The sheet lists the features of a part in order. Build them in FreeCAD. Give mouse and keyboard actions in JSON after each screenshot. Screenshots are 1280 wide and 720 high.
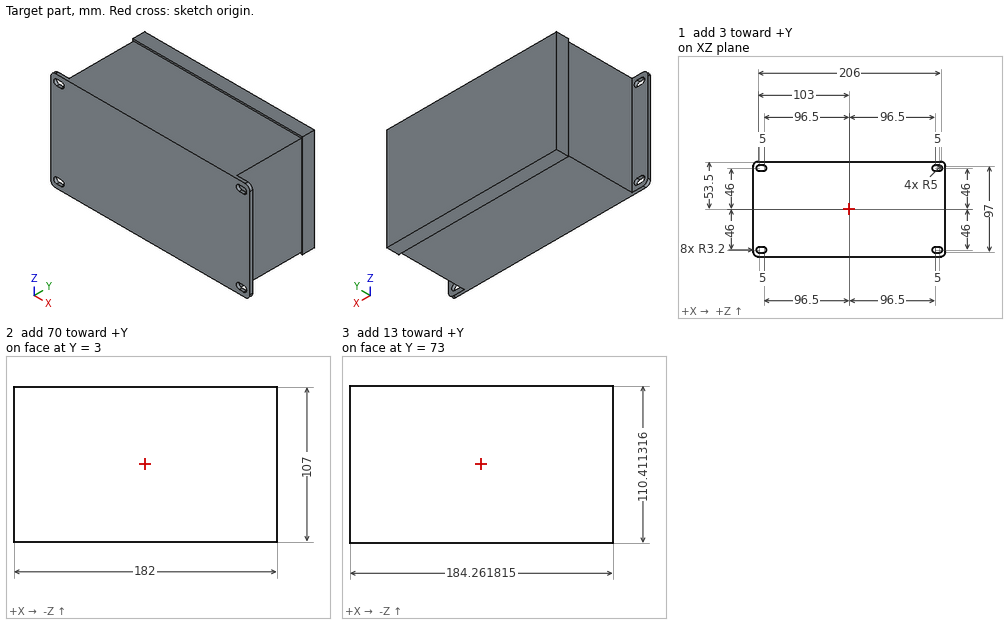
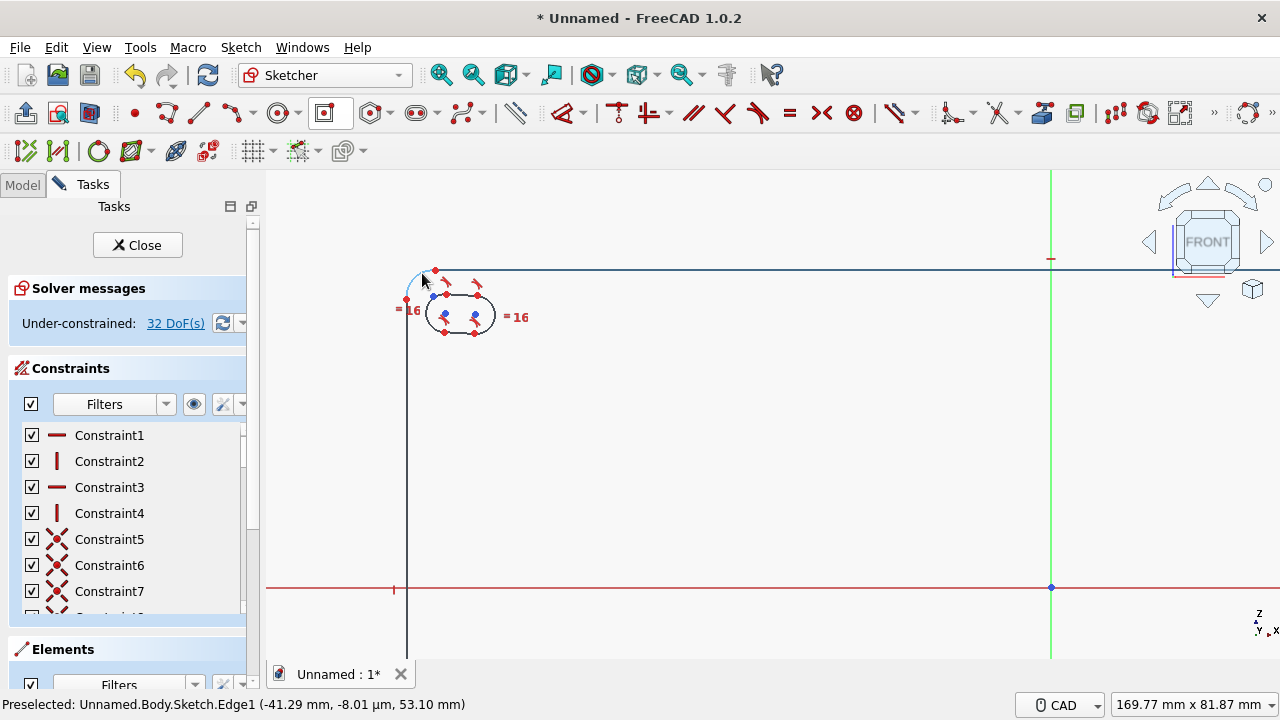
{"action": "left_click", "coordinate": [422, 273]}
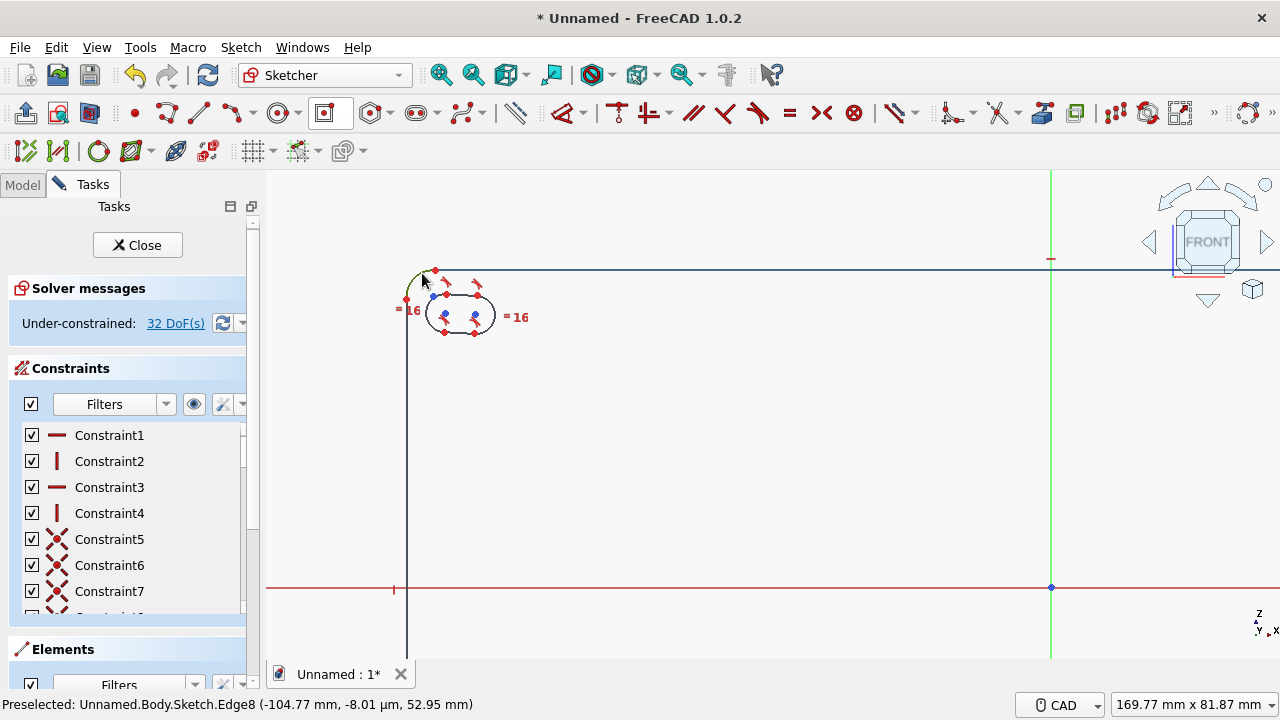
{"action": "left_click", "coordinate": [758, 114]}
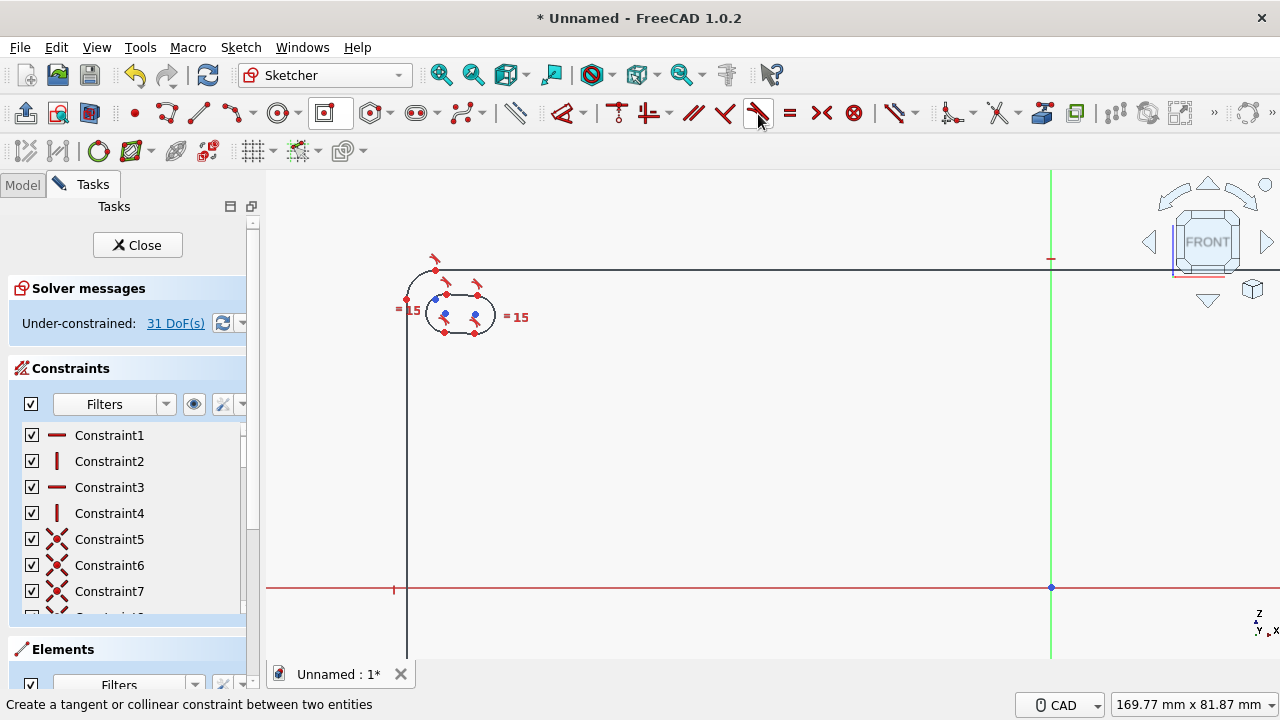
{"action": "scroll", "coordinate": [421, 273], "scroll_direction": "down", "scroll_amount": 4}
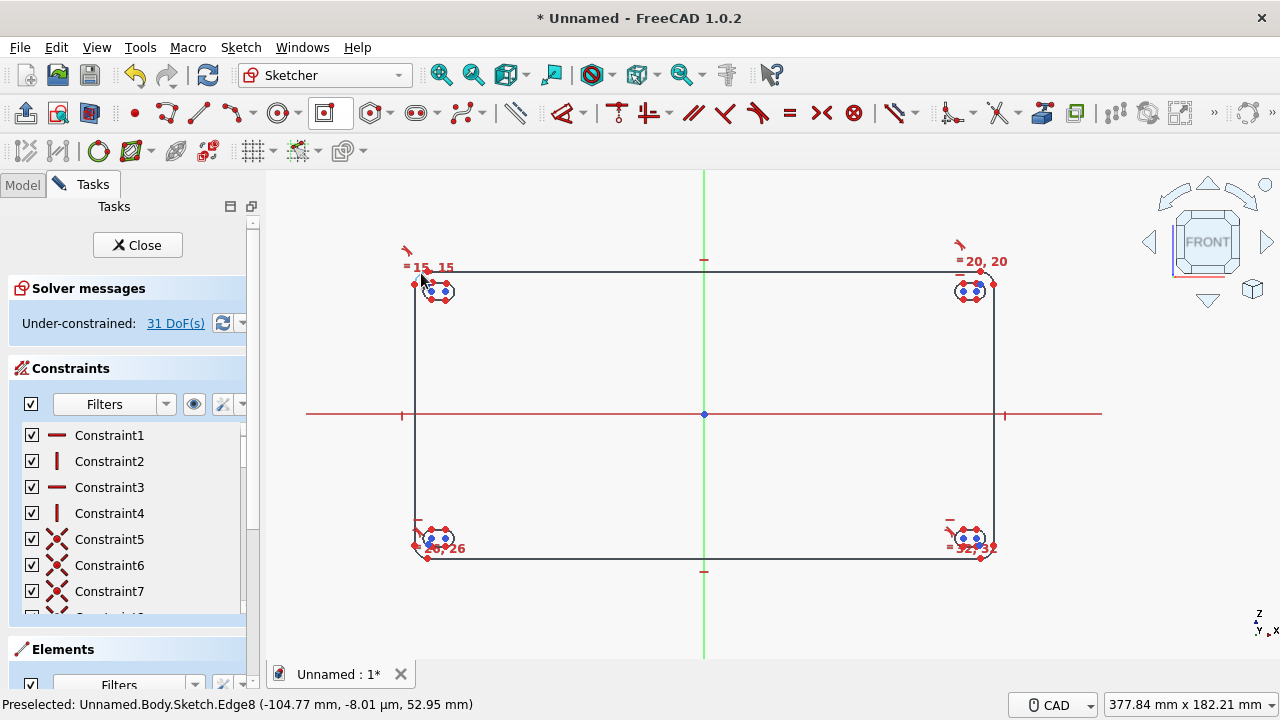
{"action": "left_click", "coordinate": [994, 363]}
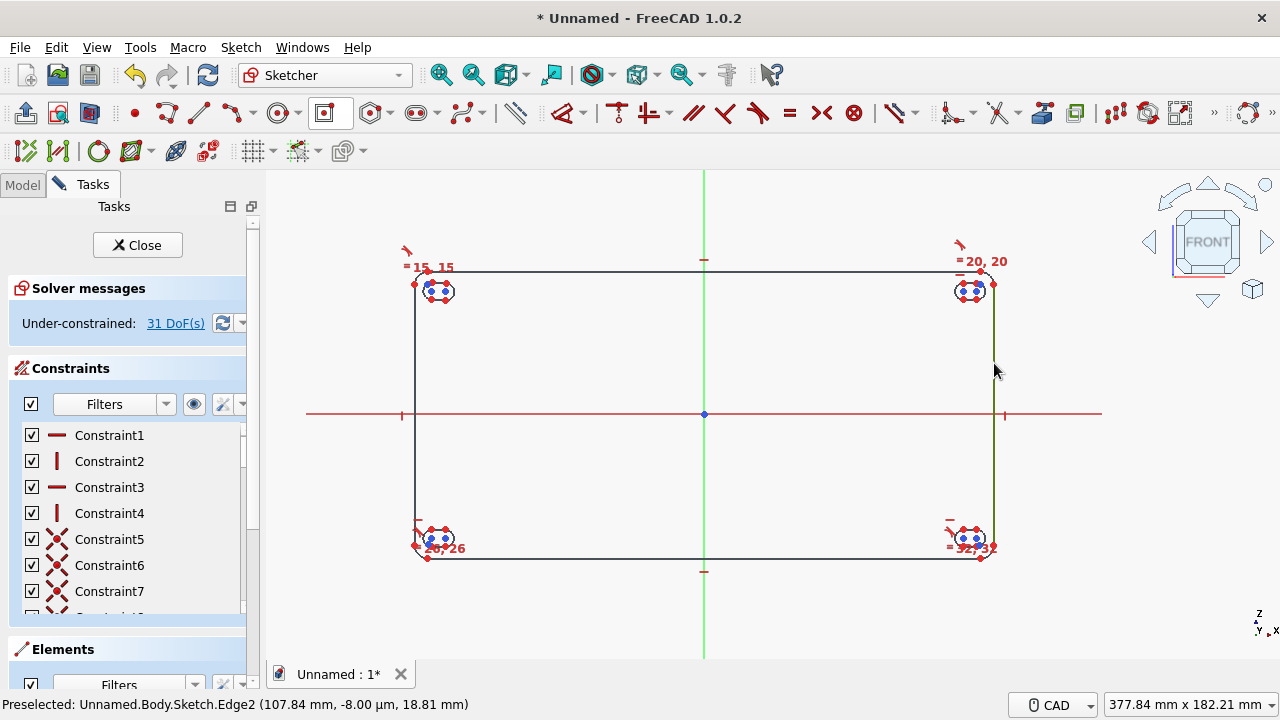
{"action": "scroll", "coordinate": [990, 276], "scroll_direction": "up", "scroll_amount": 2}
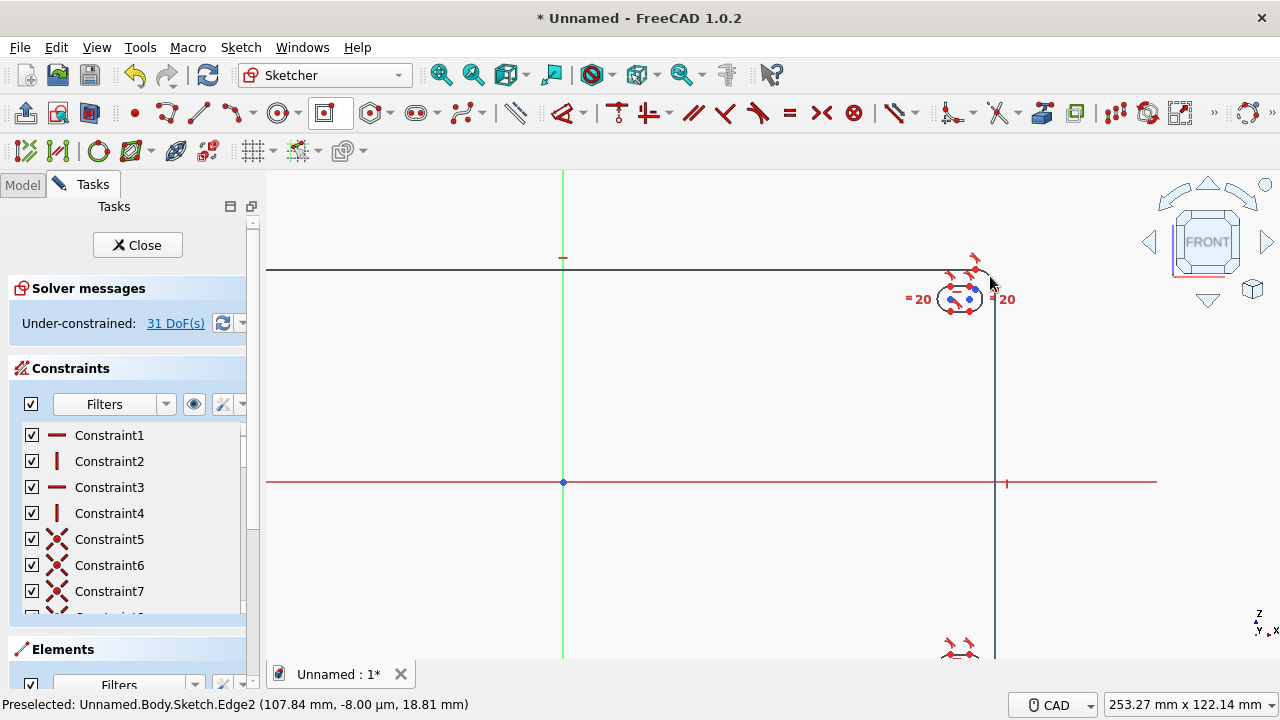
{"action": "left_click", "coordinate": [990, 276]}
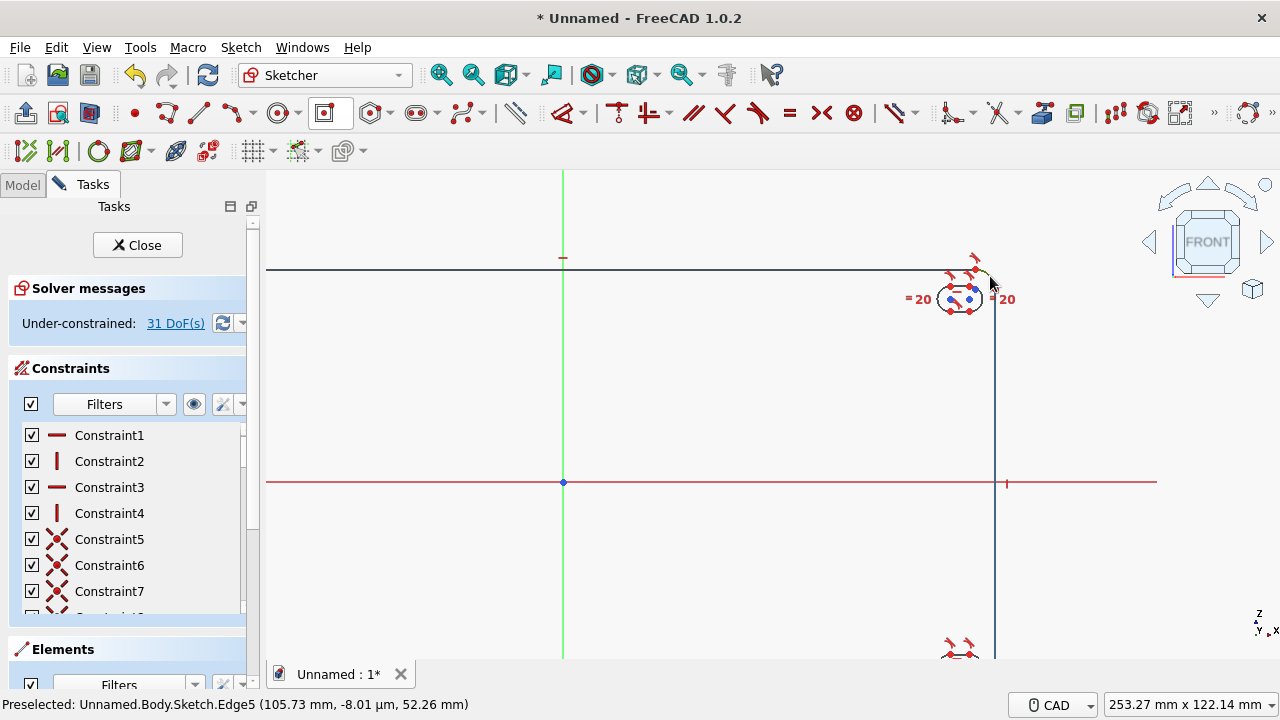
{"action": "left_click", "coordinate": [758, 114]}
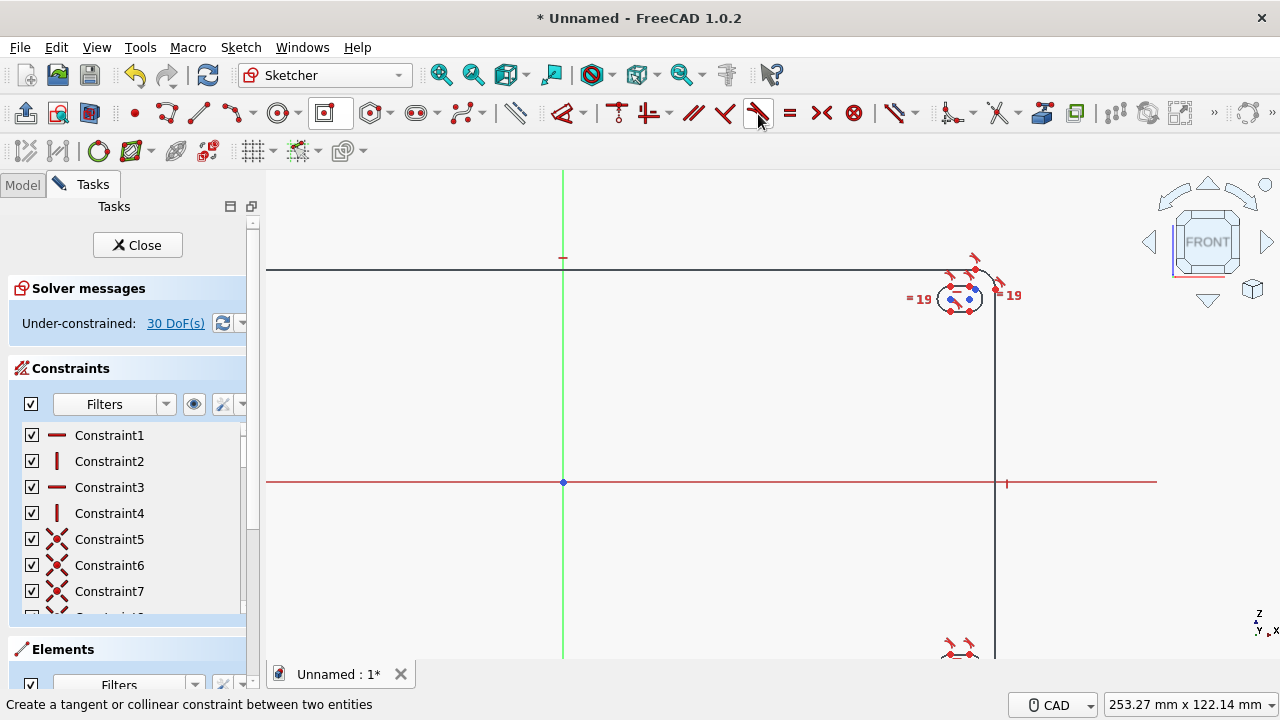
{"action": "left_click", "coordinate": [995, 406]}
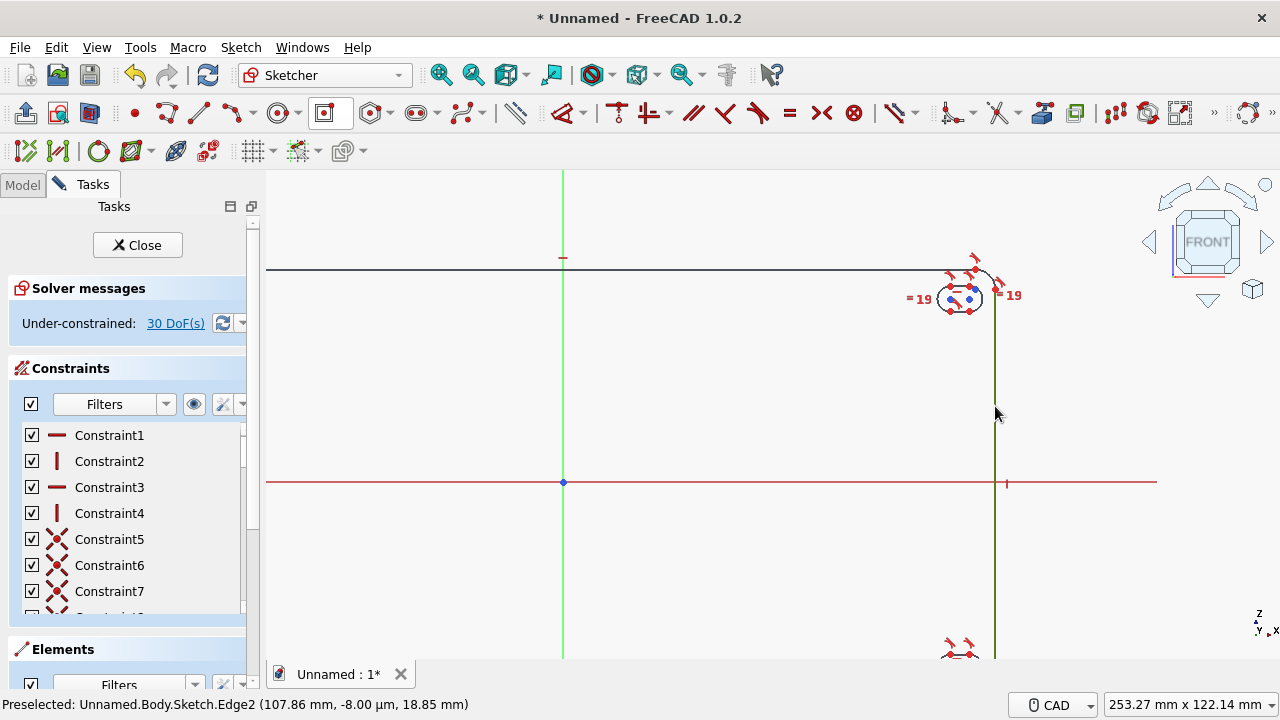
{"action": "scroll", "coordinate": [991, 276], "scroll_direction": "down", "scroll_amount": 2}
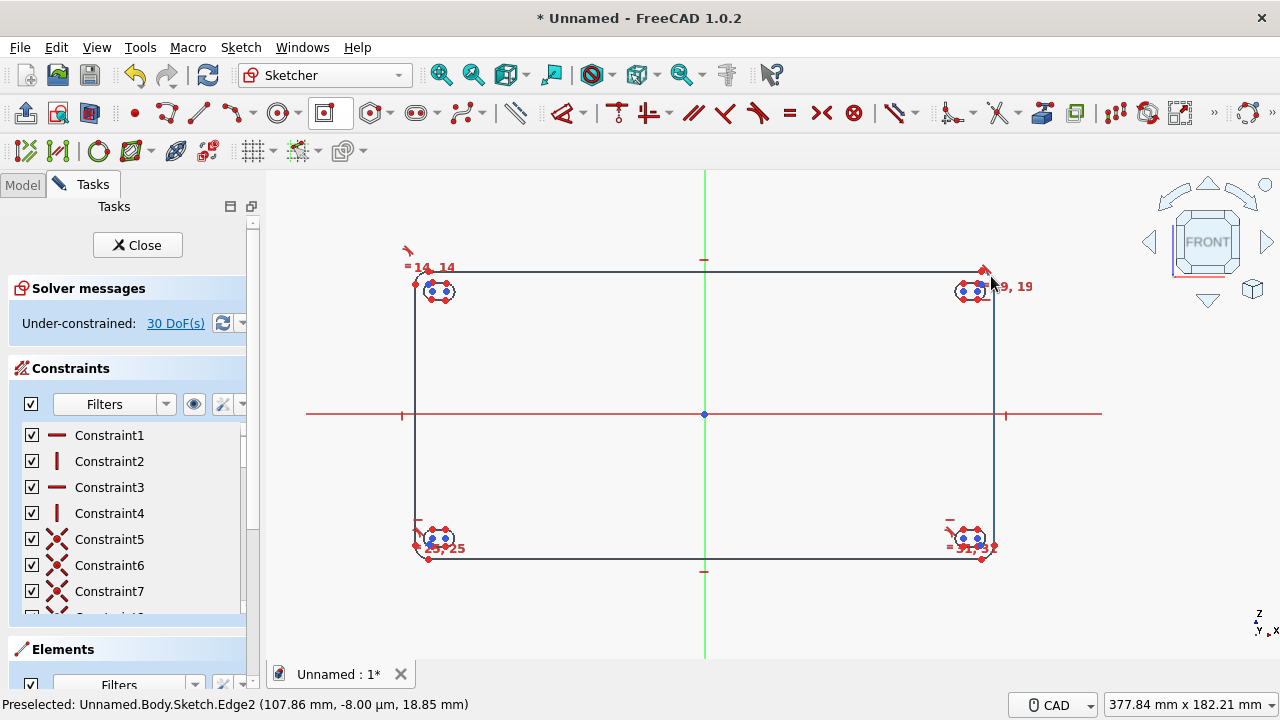
{"action": "scroll", "coordinate": [990, 555], "scroll_direction": "up", "scroll_amount": 2}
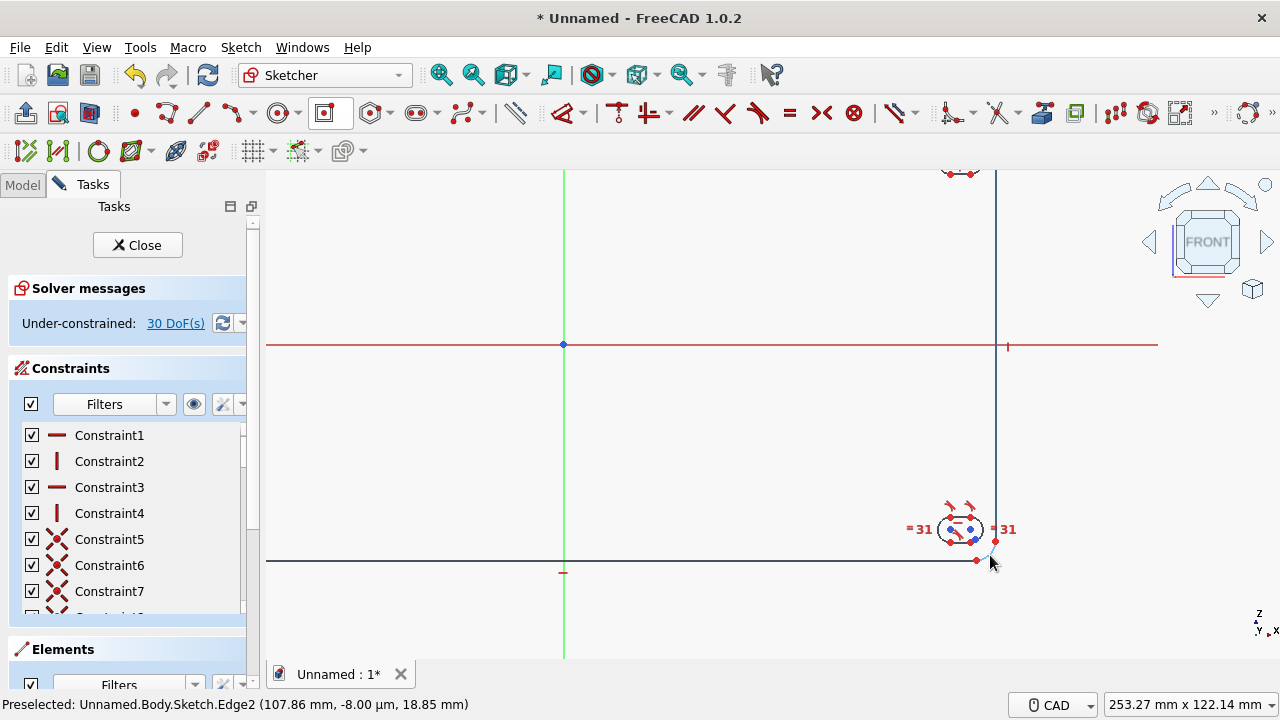
{"action": "left_click", "coordinate": [990, 555]}